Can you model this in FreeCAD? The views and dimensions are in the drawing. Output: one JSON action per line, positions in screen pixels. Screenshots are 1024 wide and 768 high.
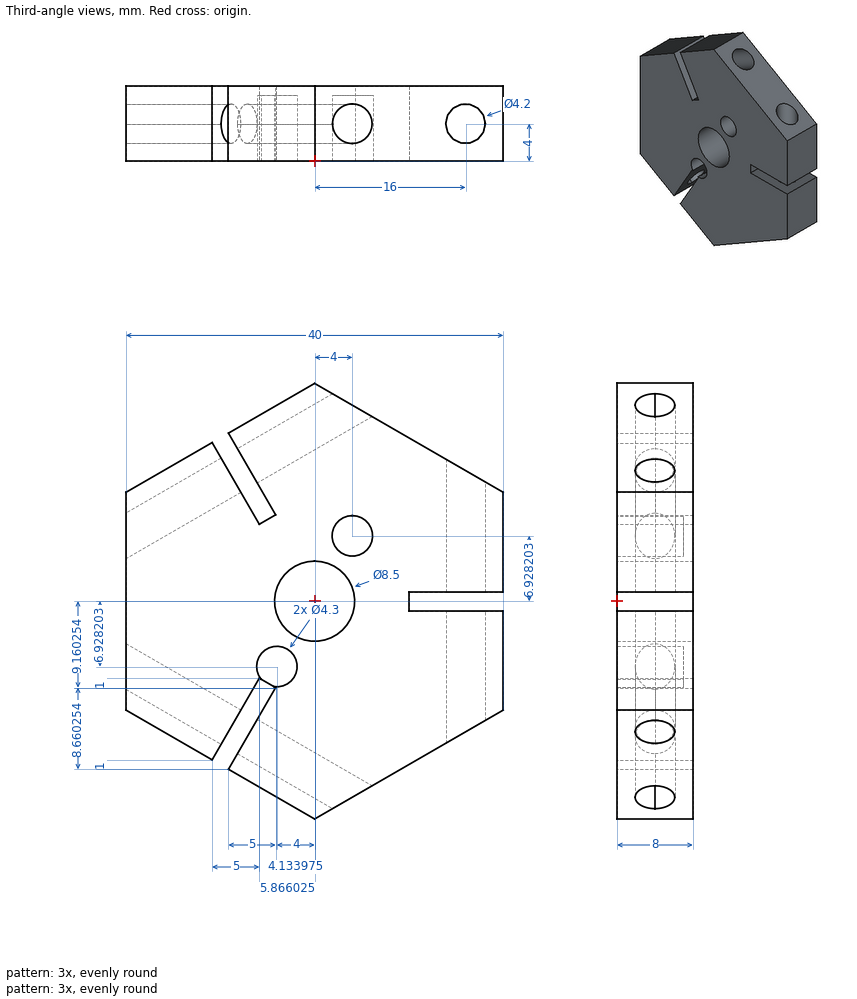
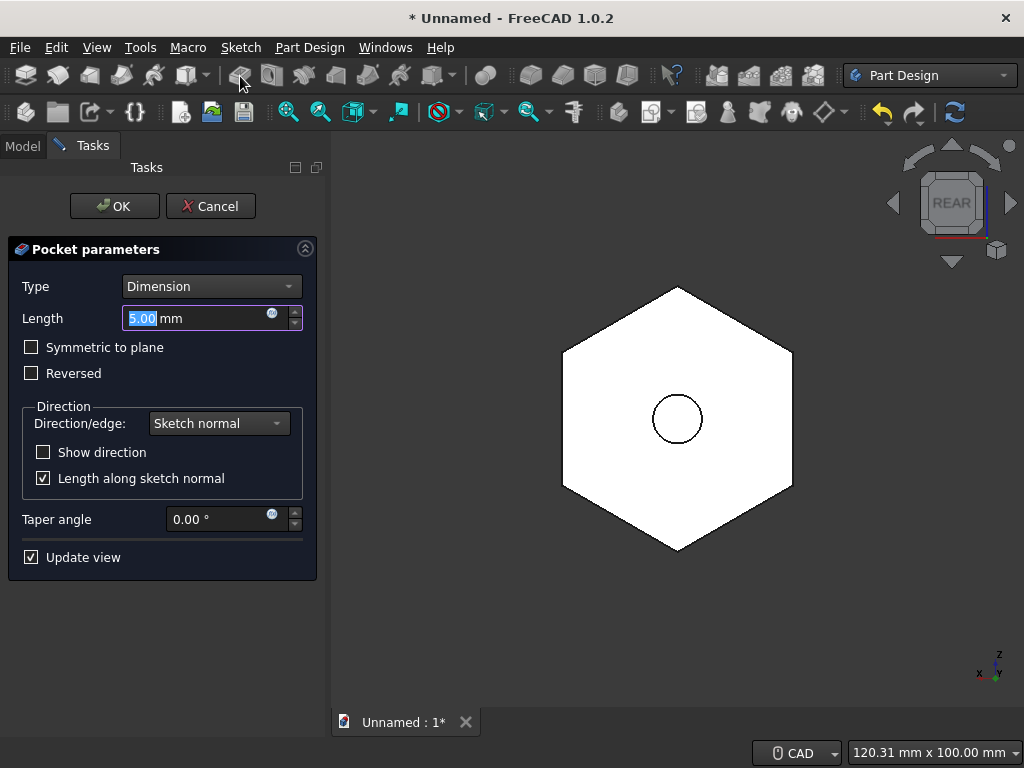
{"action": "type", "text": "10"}
{"action": "key", "text": "Tab"}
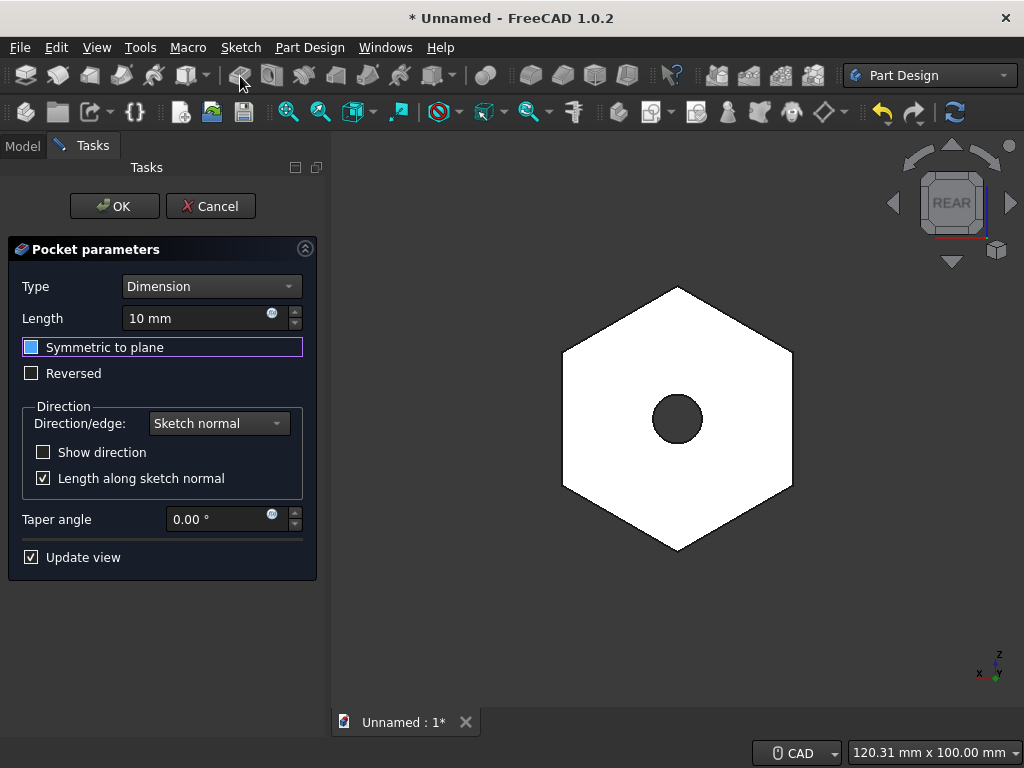
{"action": "left_click", "coordinate": [115, 206]}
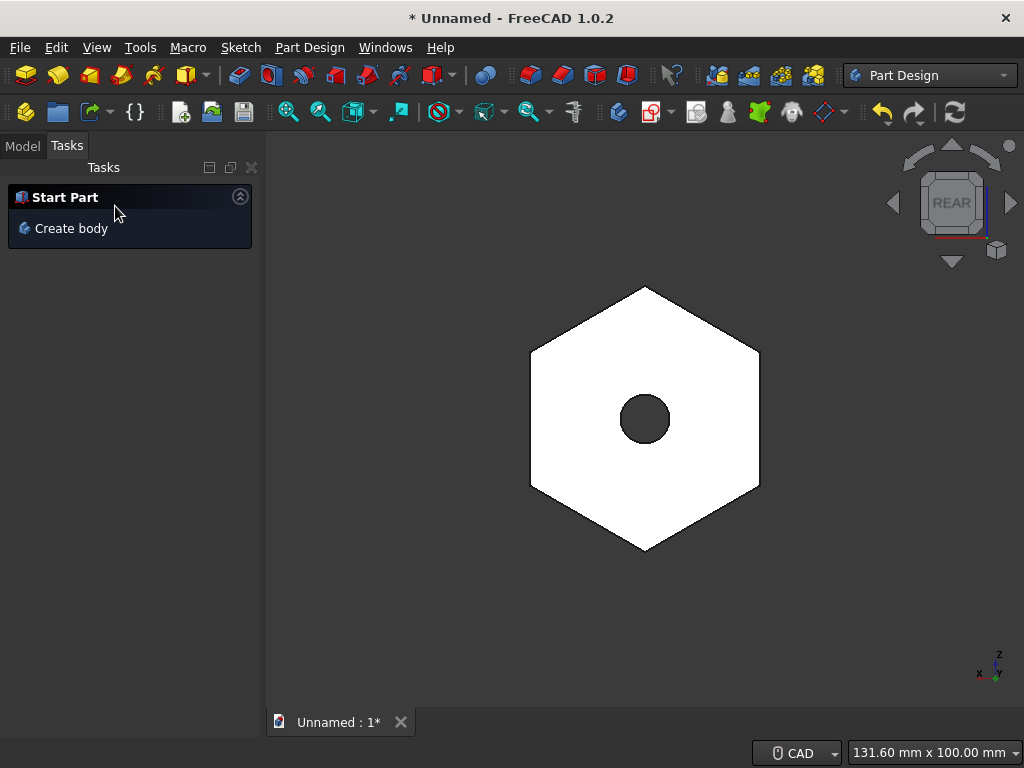
{"action": "left_click", "coordinate": [579, 380]}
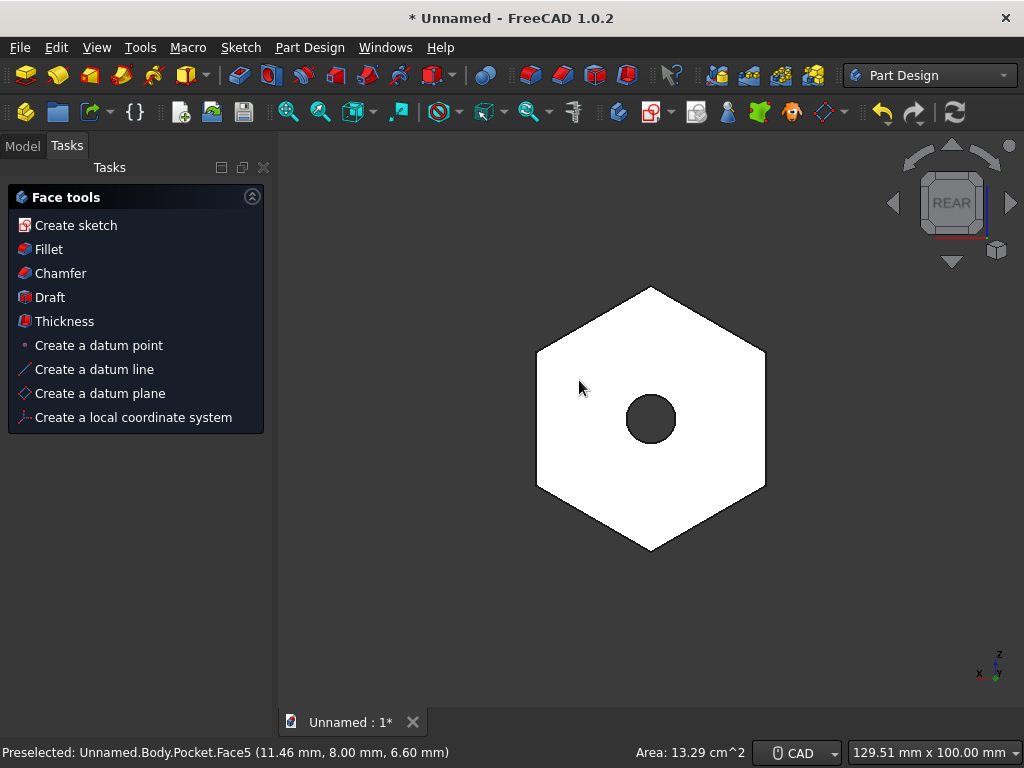
{"action": "left_click", "coordinate": [652, 112]}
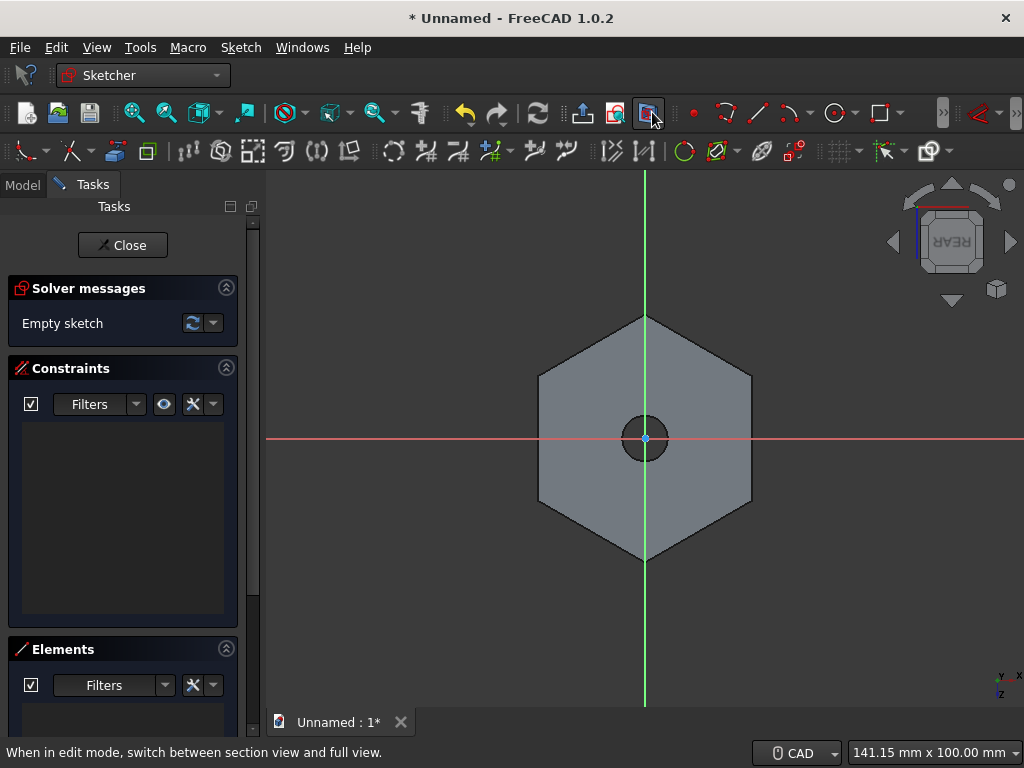
{"action": "scroll", "coordinate": [633, 370], "scroll_direction": "up", "scroll_amount": 6}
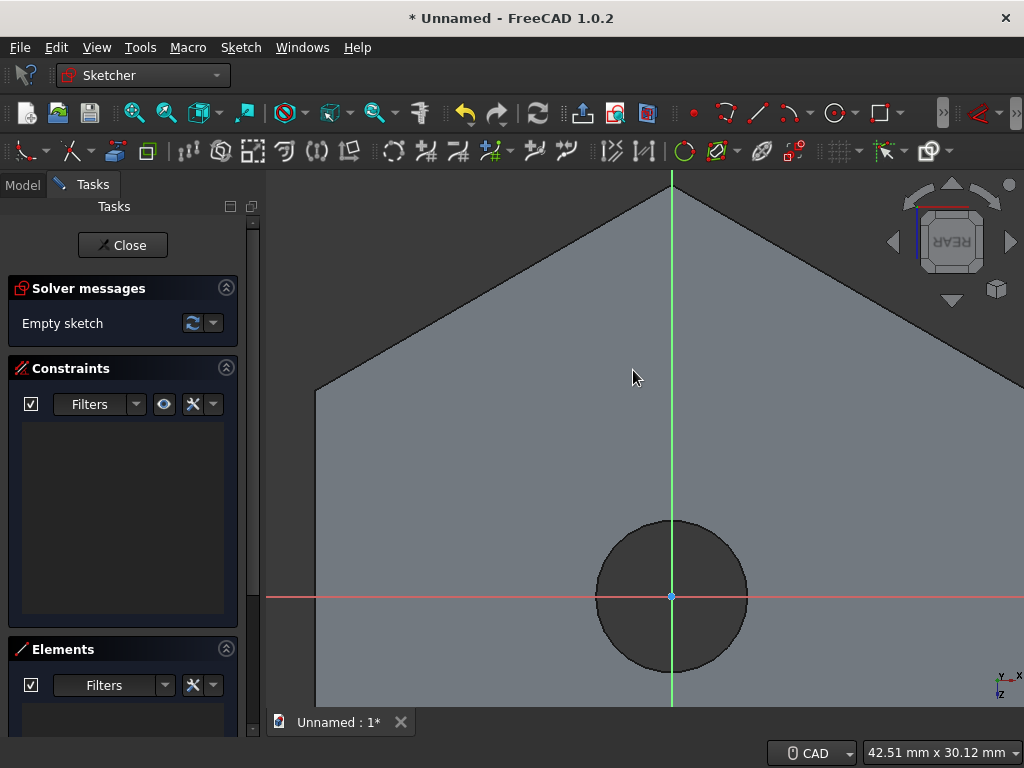
{"action": "left_click", "coordinate": [726, 114]}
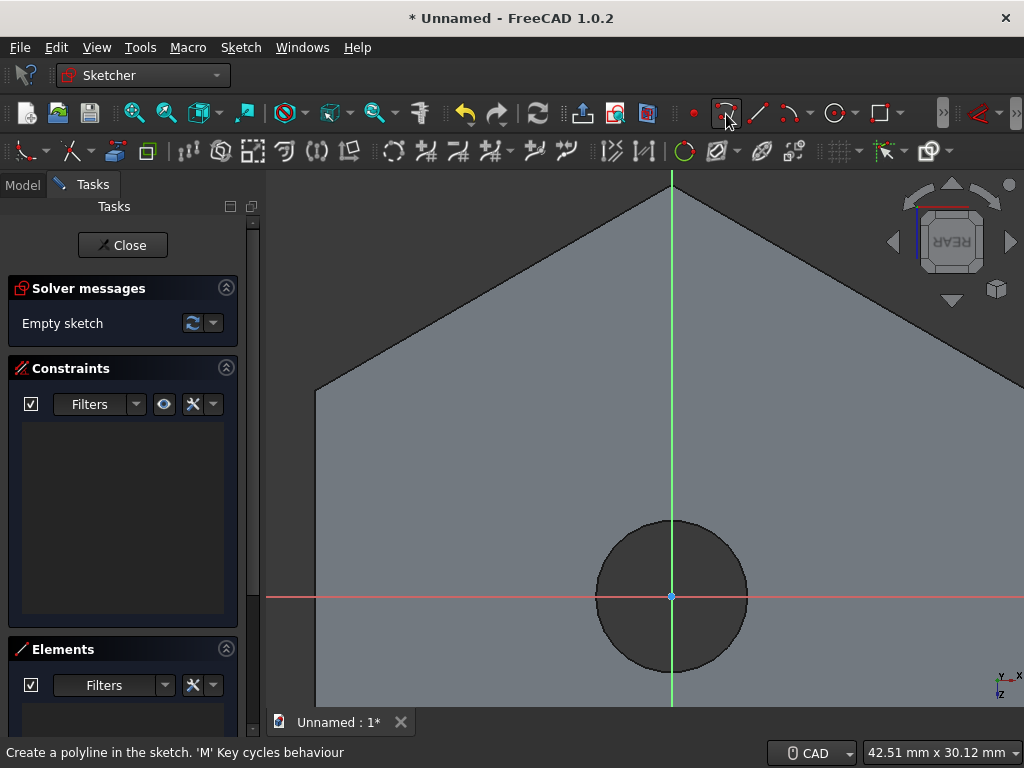
{"action": "left_click", "coordinate": [598, 433]}
{"action": "left_click", "coordinate": [509, 279]}
{"action": "left_click", "coordinate": [478, 297]}
{"action": "left_click", "coordinate": [567, 451]}
{"action": "left_click", "coordinate": [598, 434]}
{"action": "key", "text": "Escape"}
{"action": "key", "text": "Escape"}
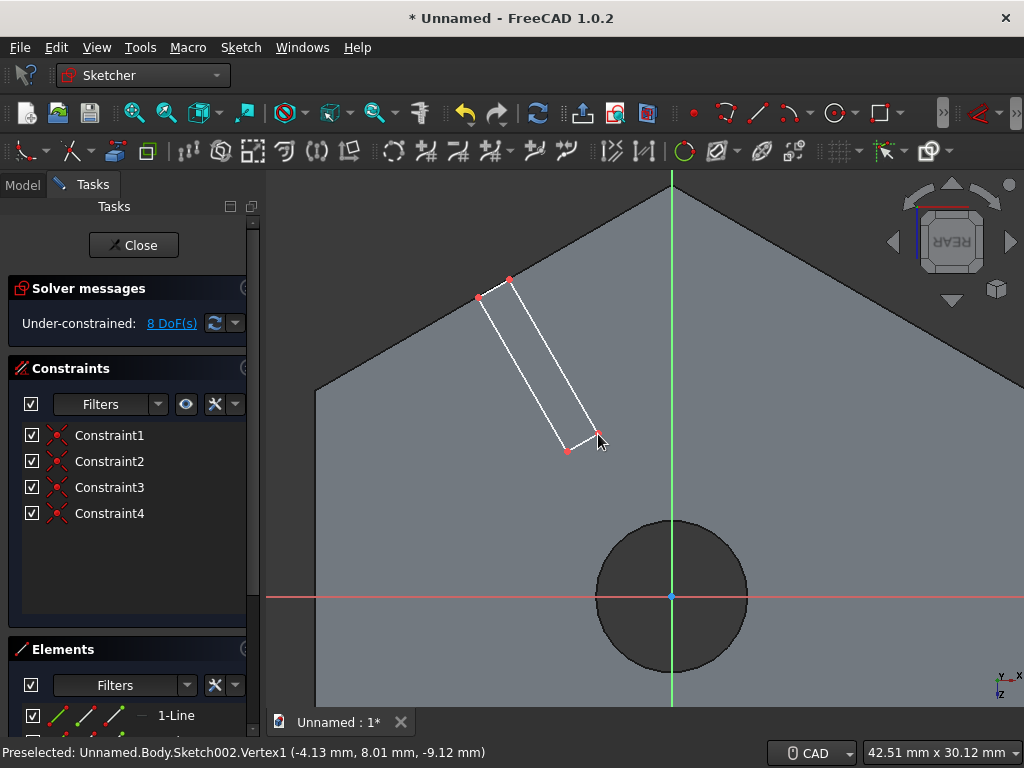
{"action": "left_click", "coordinate": [978, 114]}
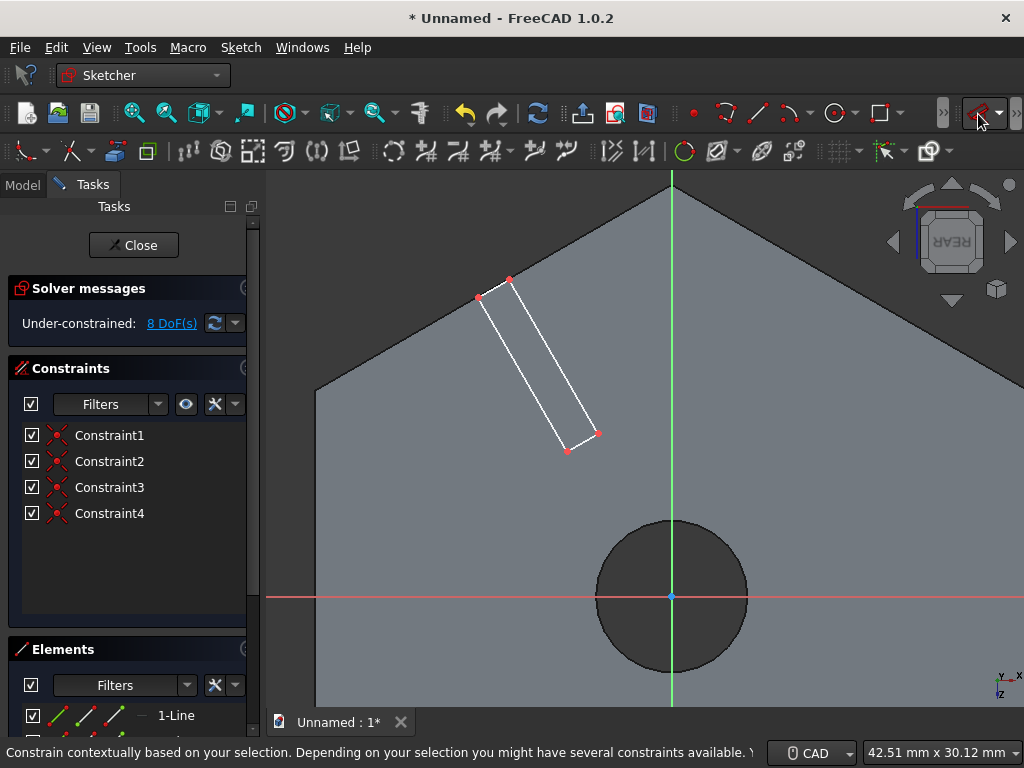
{"action": "left_click", "coordinate": [571, 388]}
{"action": "left_click", "coordinate": [553, 246]}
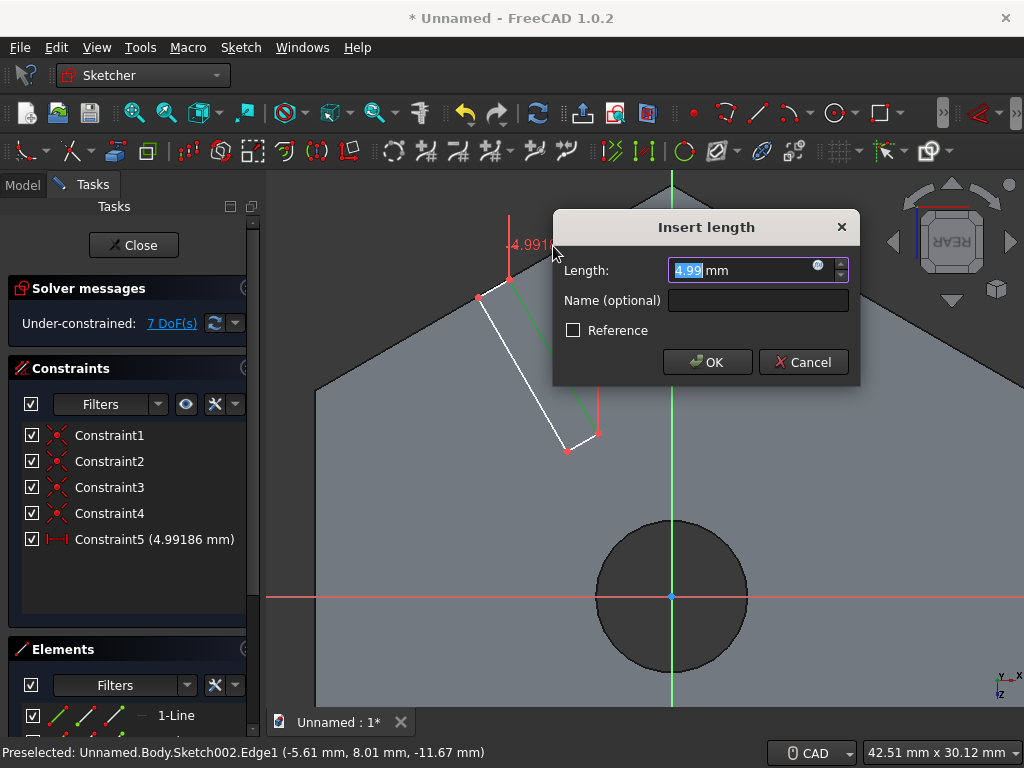
{"action": "type", "text": "5"}
{"action": "key", "text": "Return"}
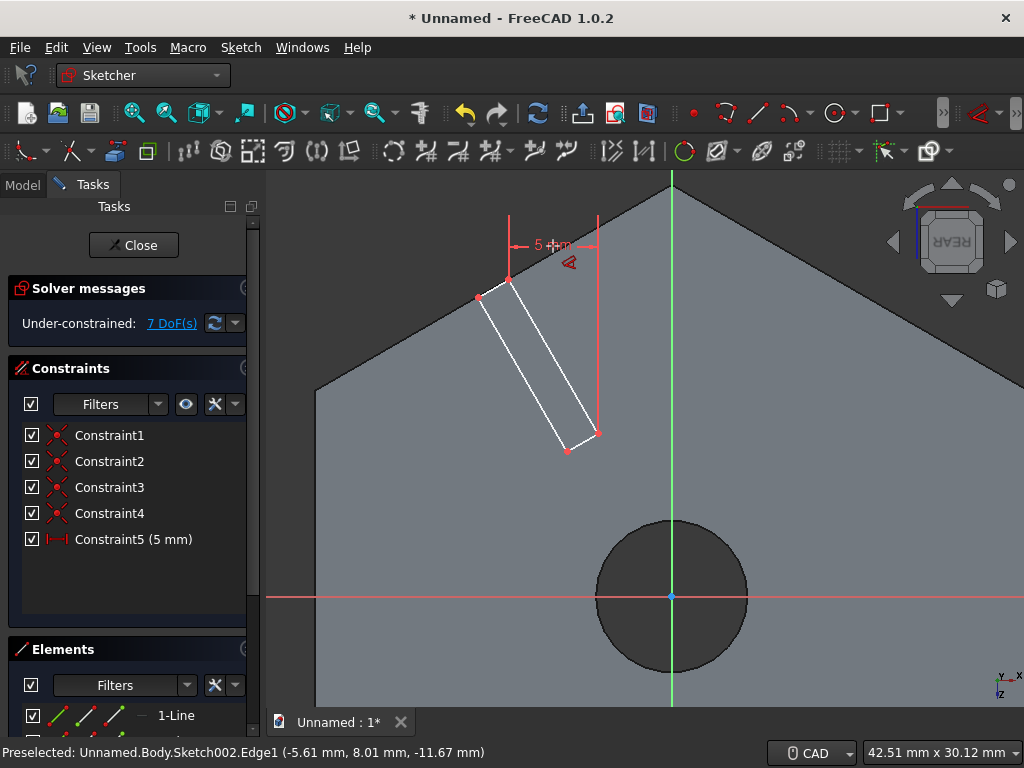
{"action": "scroll", "coordinate": [500, 285], "scroll_direction": "up", "scroll_amount": 5}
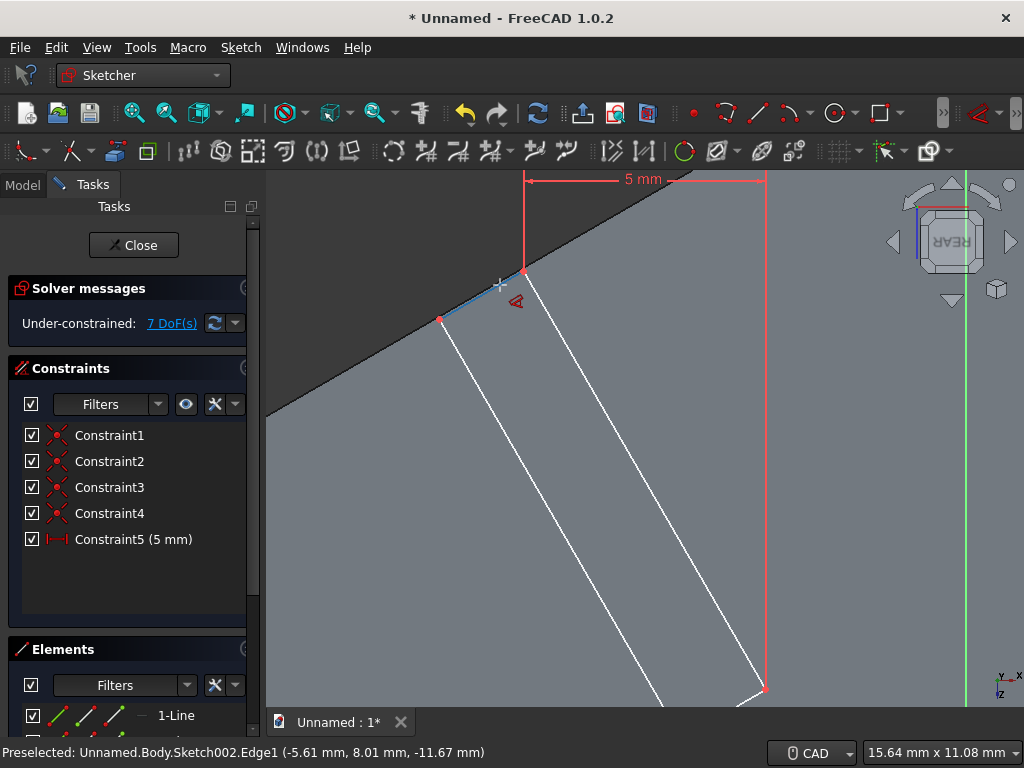
{"action": "left_click", "coordinate": [498, 286]}
{"action": "left_click", "coordinate": [406, 296]}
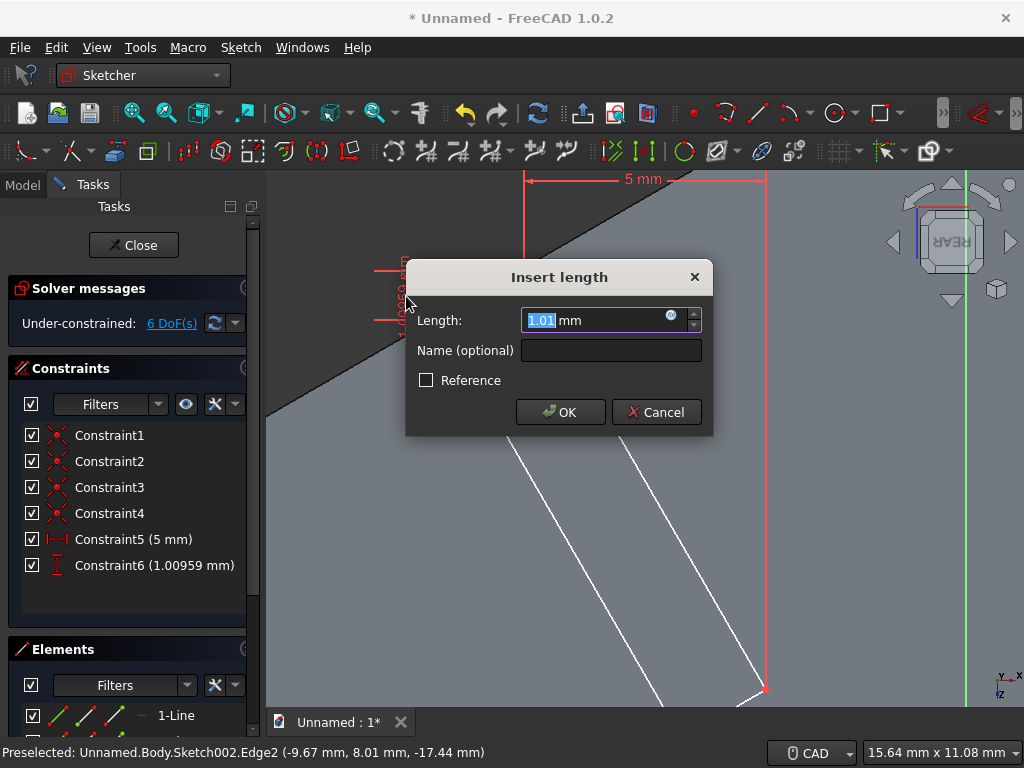
{"action": "type", "text": "1"}
{"action": "key", "text": "Return"}